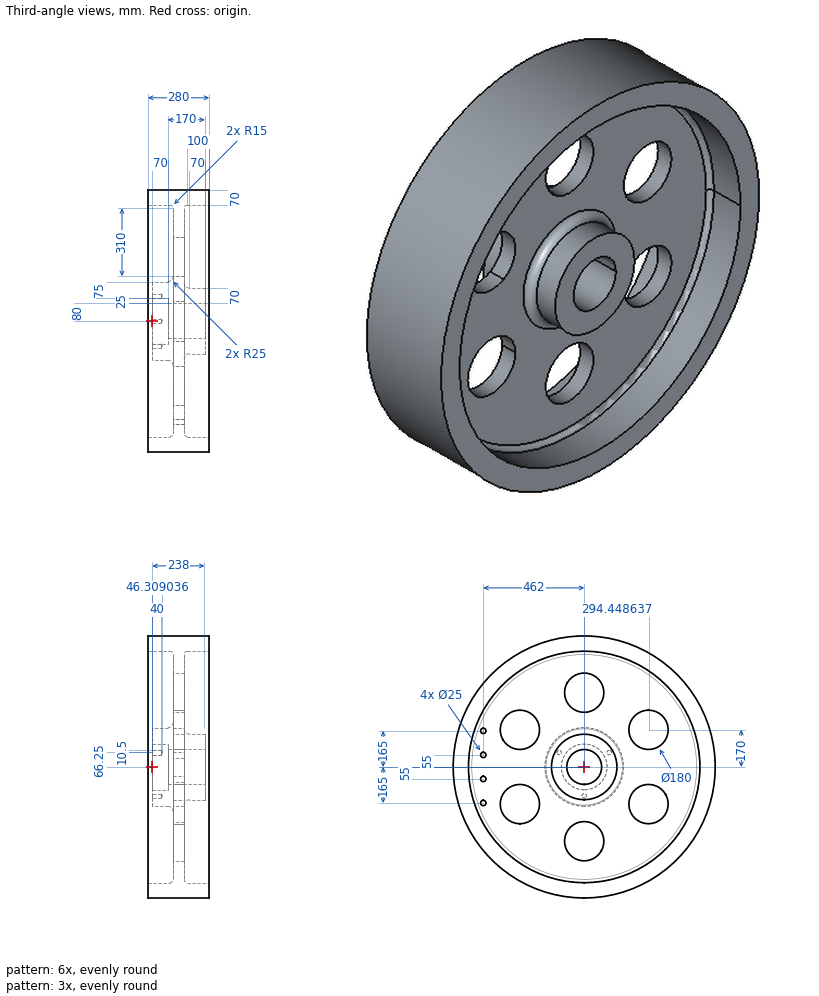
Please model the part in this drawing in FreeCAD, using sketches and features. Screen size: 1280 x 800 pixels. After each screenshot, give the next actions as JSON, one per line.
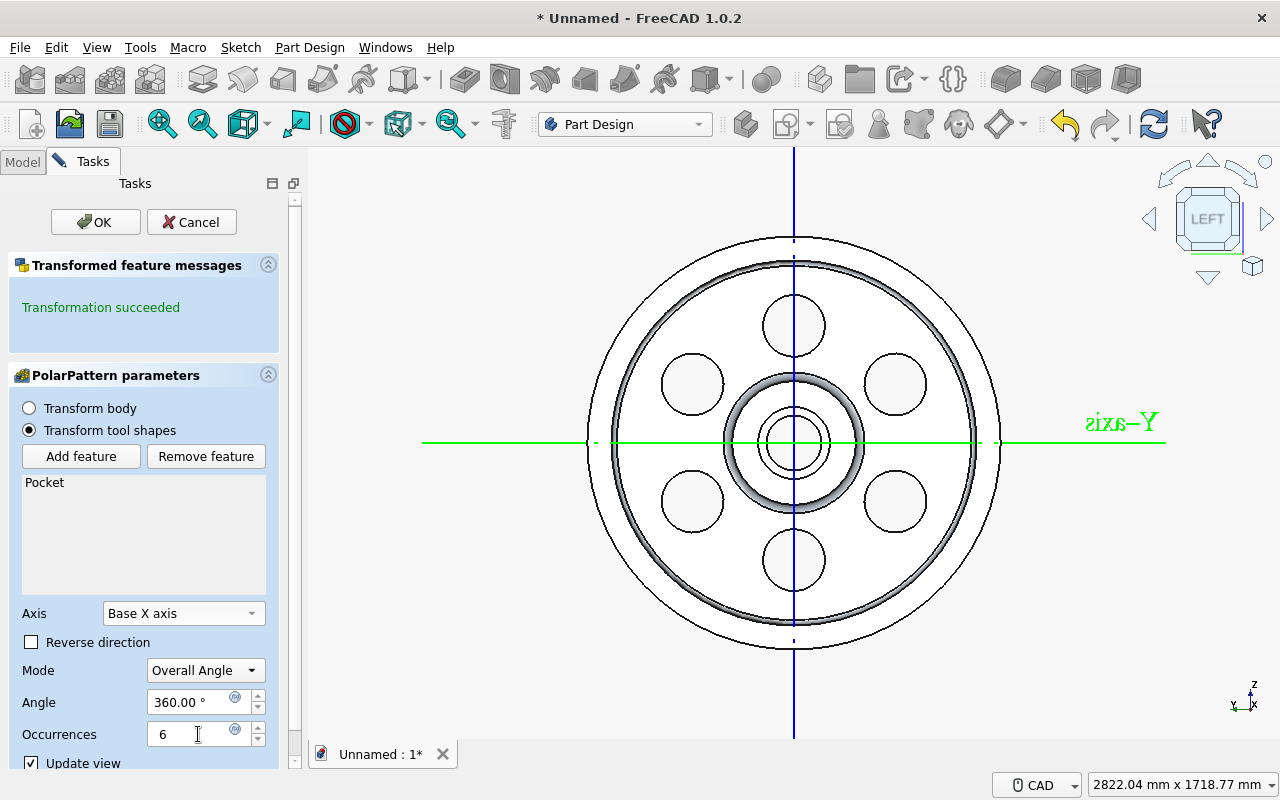
{"action": "left_click", "coordinate": [96, 222]}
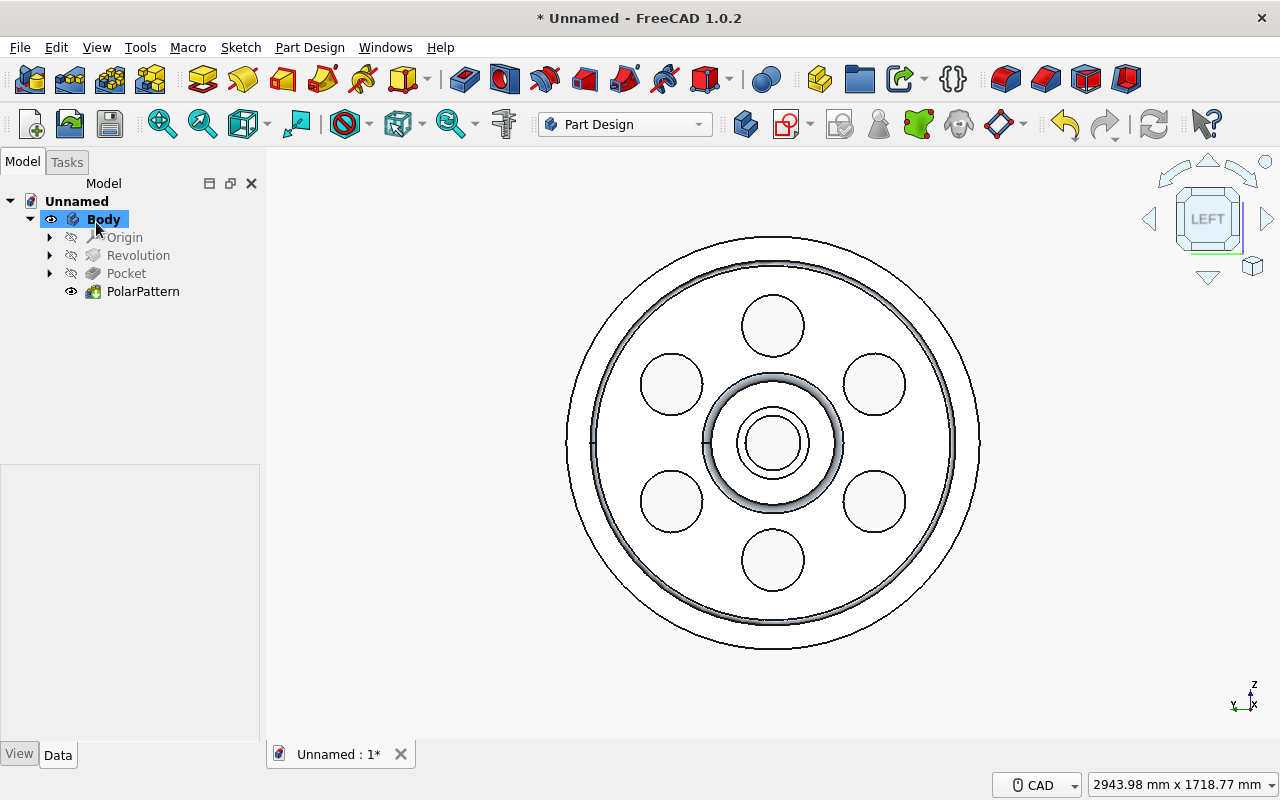
{"action": "left_click", "coordinate": [50, 237]}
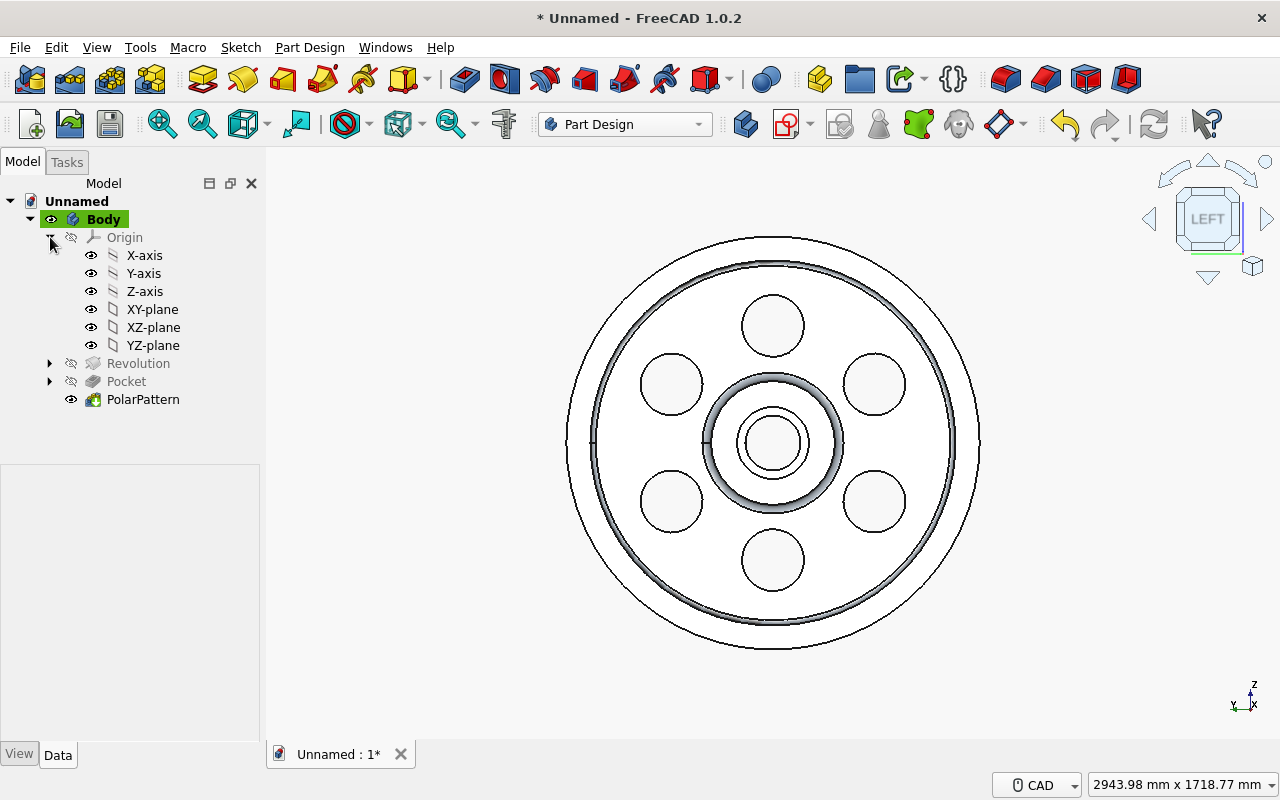
{"action": "left_click", "coordinate": [136, 327]}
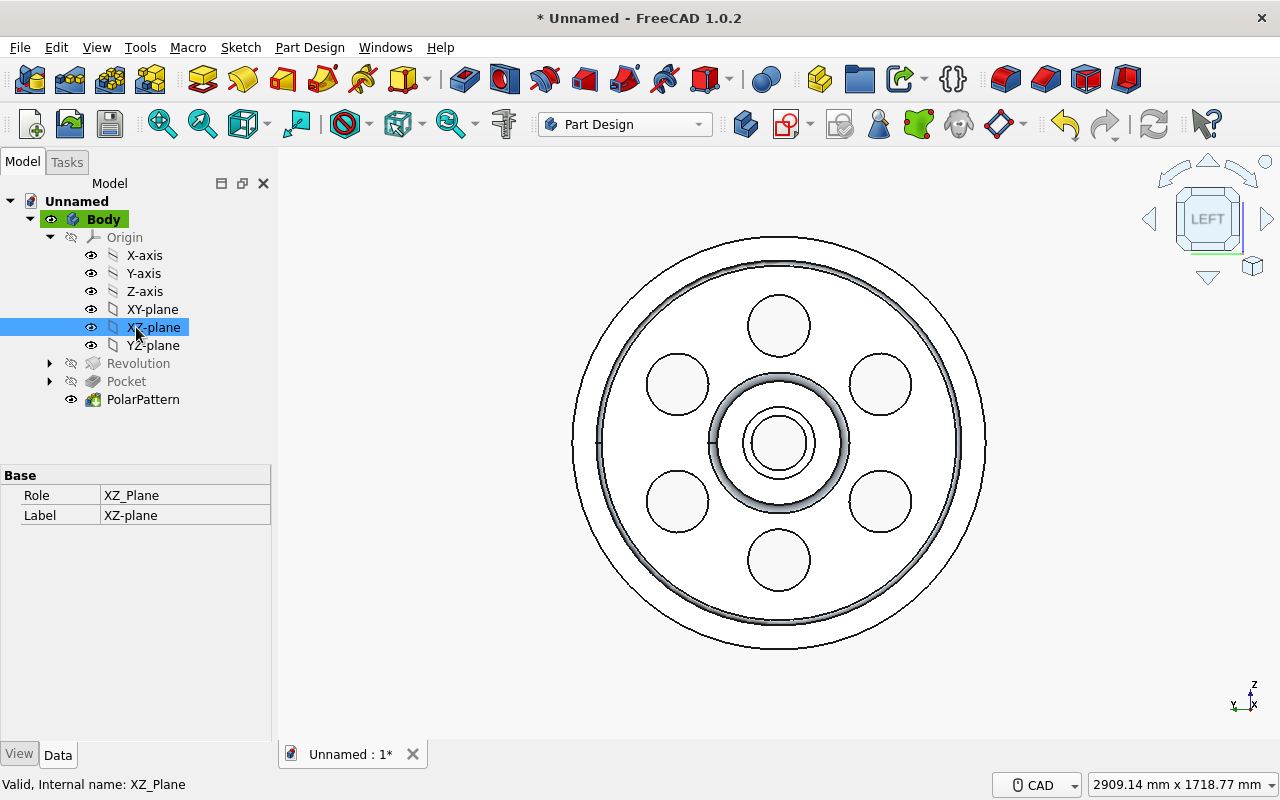
{"action": "left_click", "coordinate": [1000, 124]}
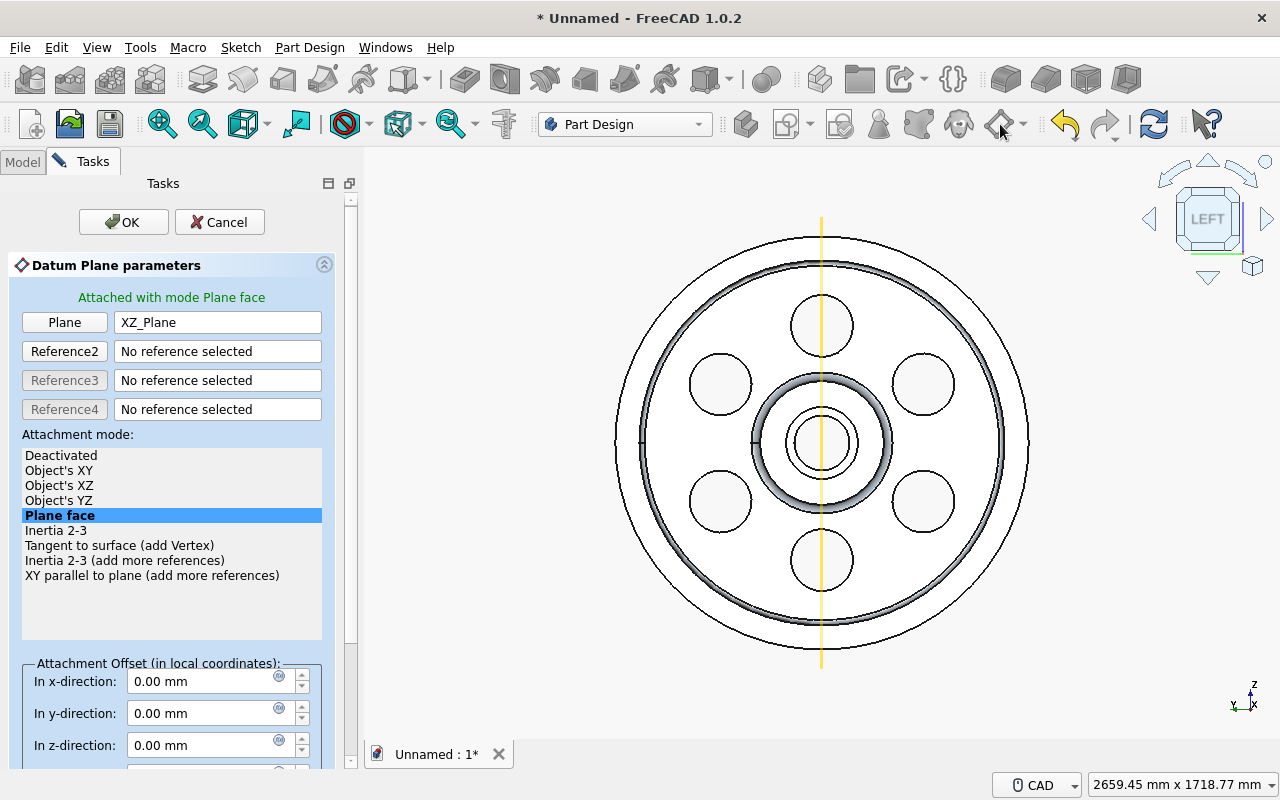
{"action": "triple_click", "coordinate": [210, 745]}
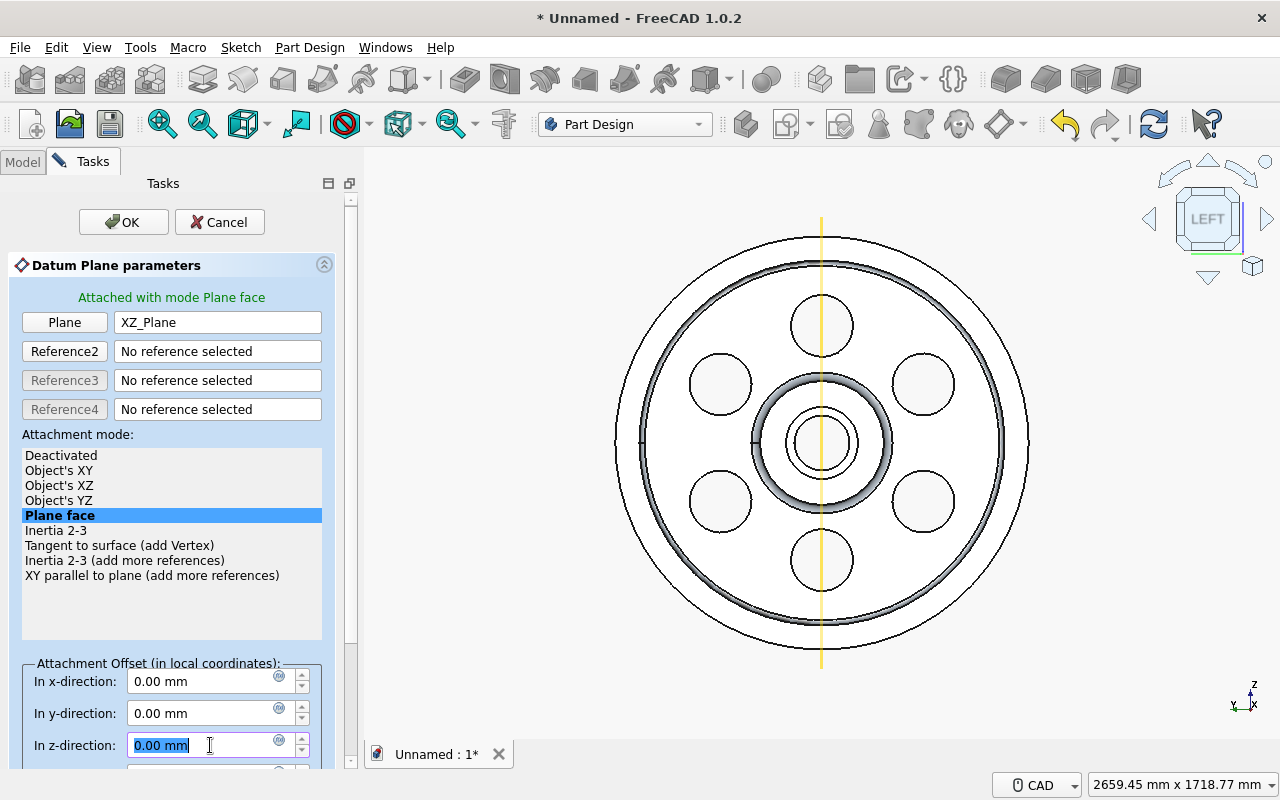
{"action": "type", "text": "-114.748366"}
{"action": "key", "text": "Tab"}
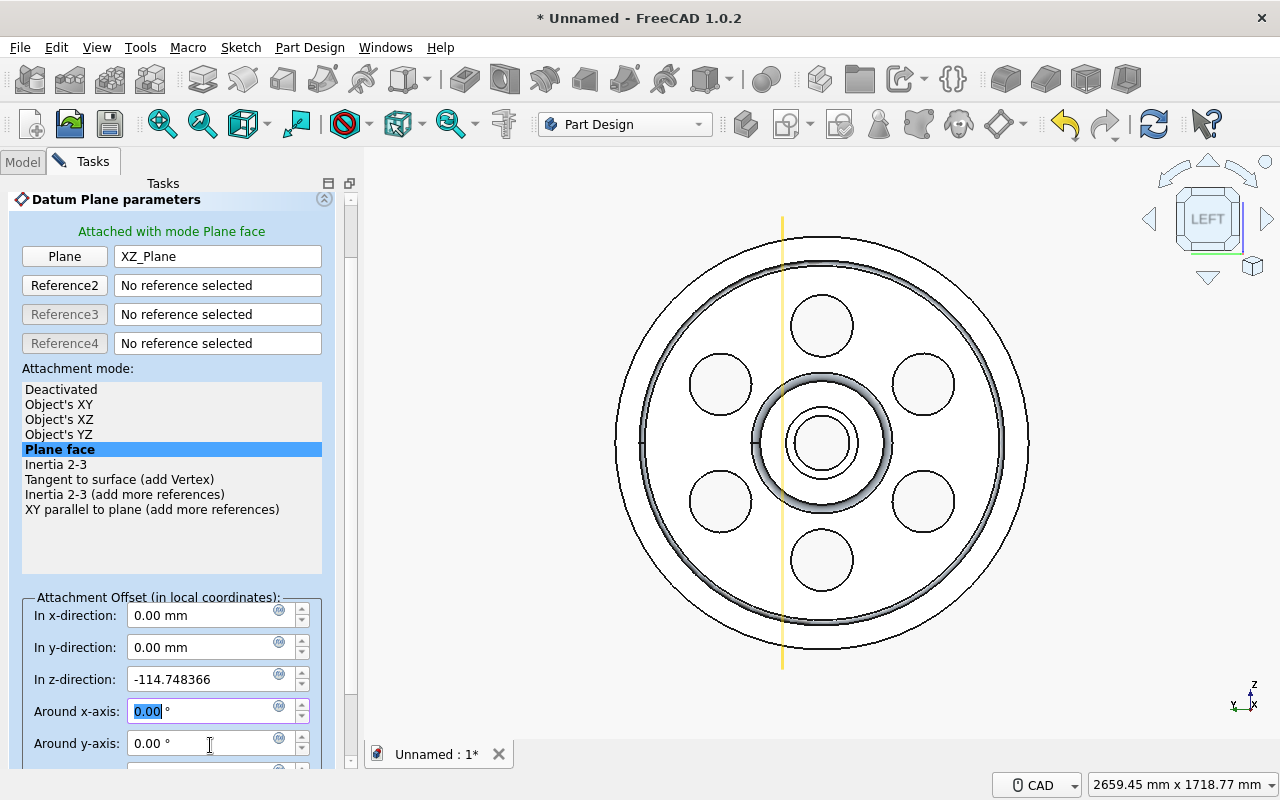
{"action": "scroll", "coordinate": [351, 480], "scroll_direction": "up", "scroll_amount": 2}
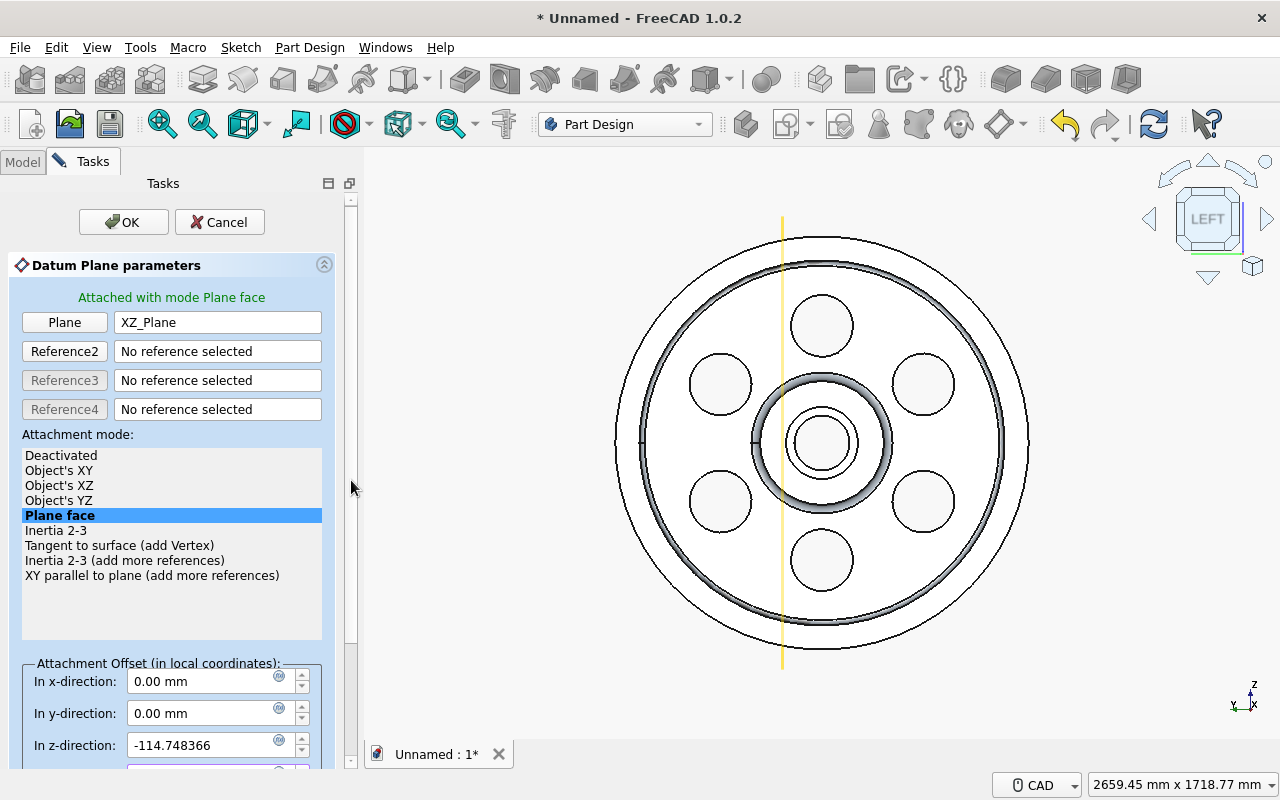
{"action": "left_click", "coordinate": [124, 222]}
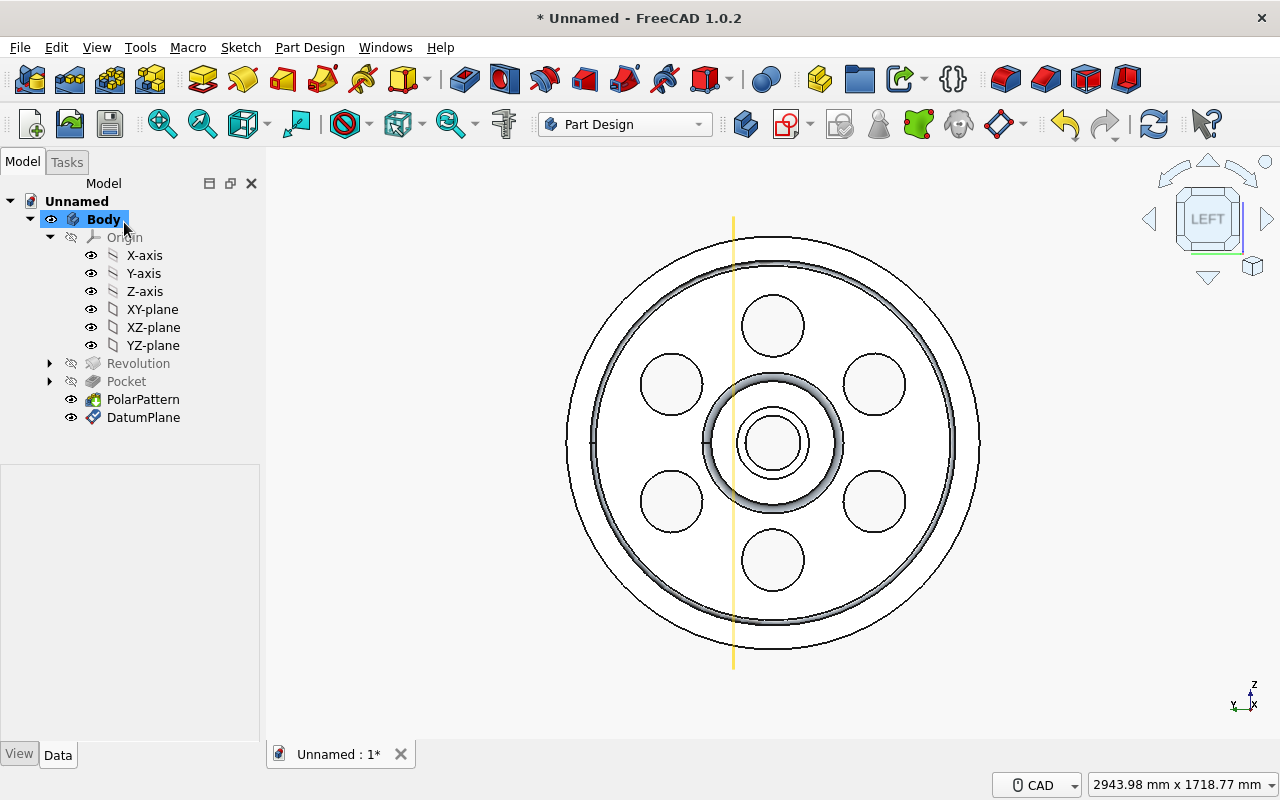
{"action": "left_click", "coordinate": [116, 417]}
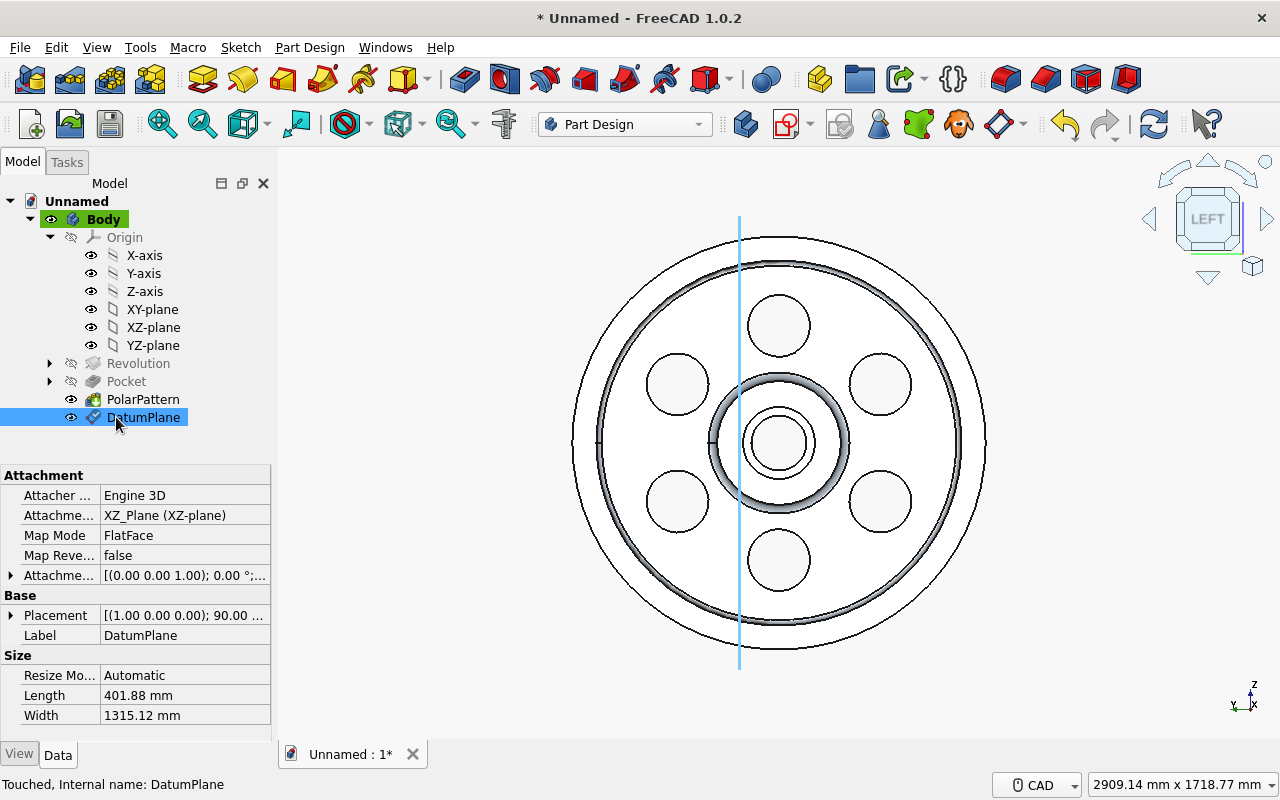
{"action": "left_click", "coordinate": [786, 124]}